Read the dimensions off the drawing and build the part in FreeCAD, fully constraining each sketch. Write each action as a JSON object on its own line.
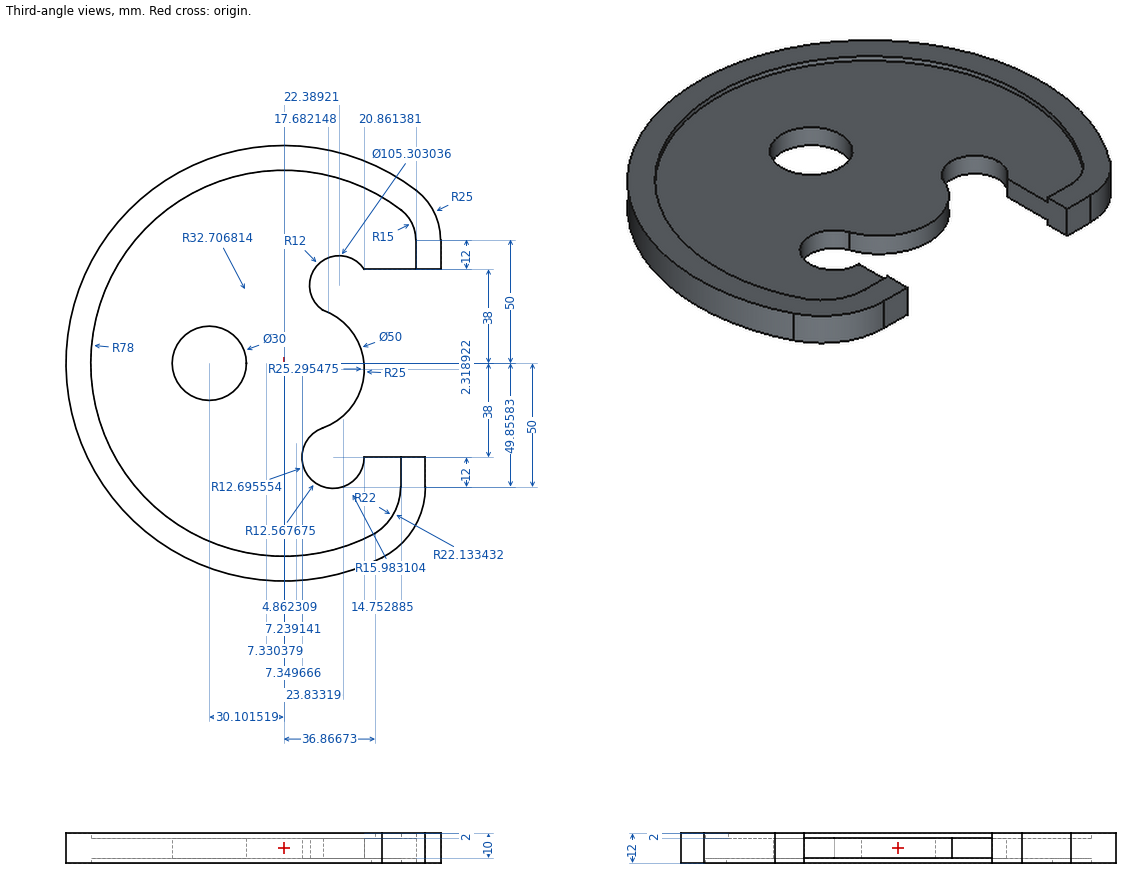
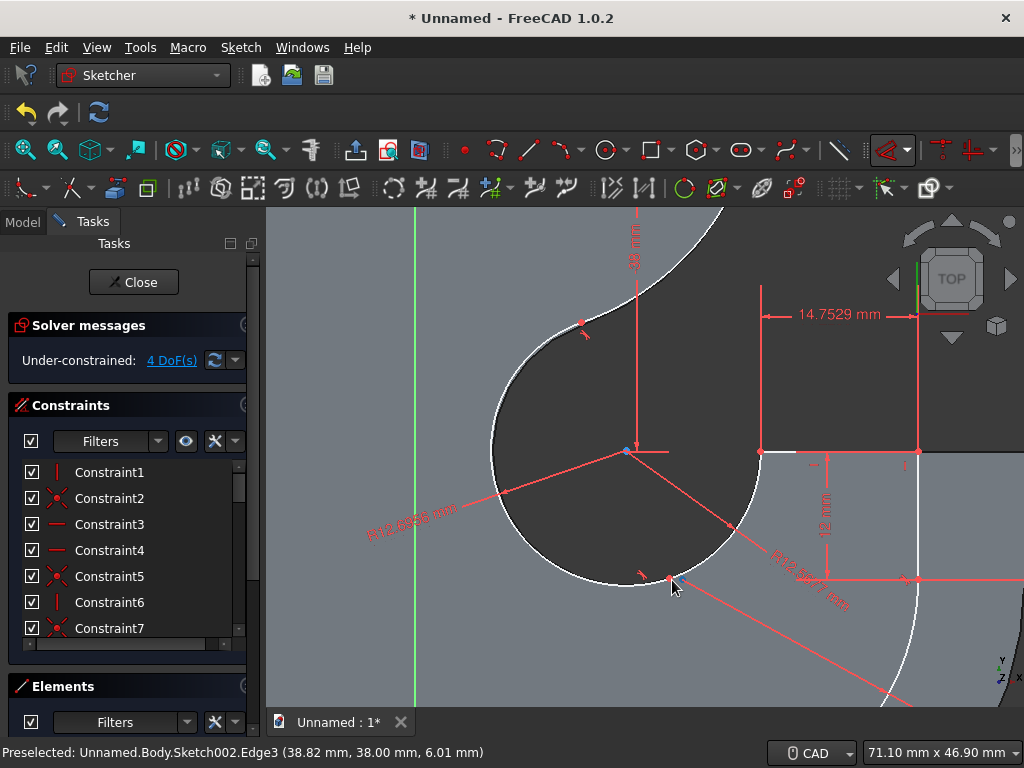
{"action": "left_click", "coordinate": [670, 579]}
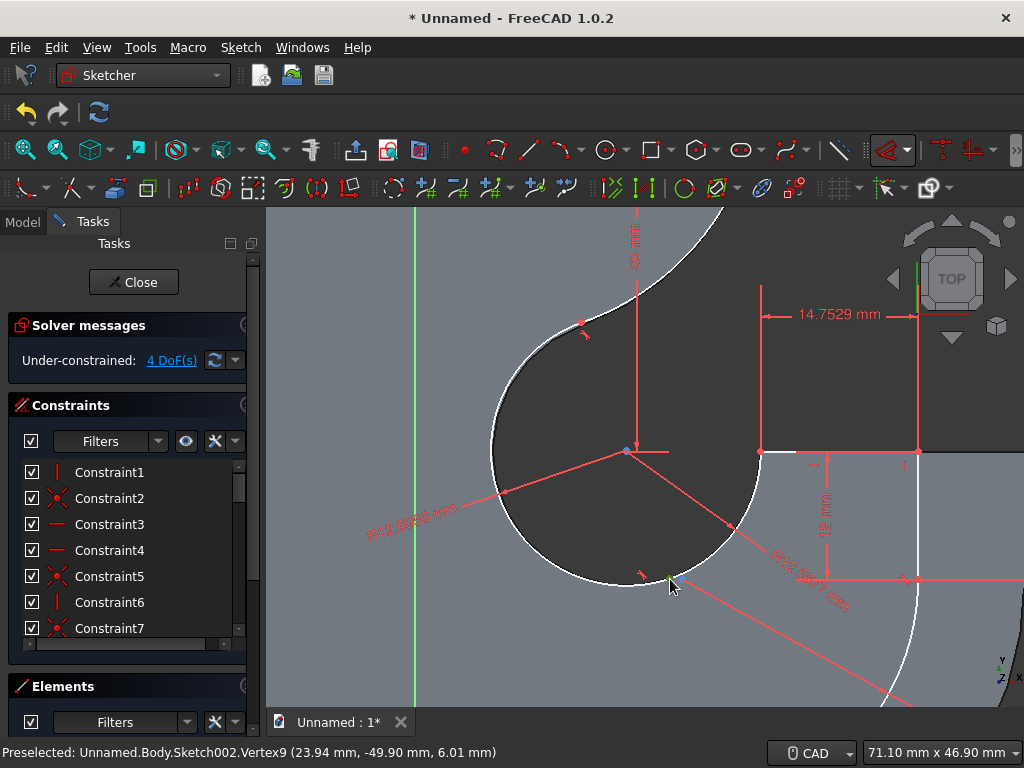
{"action": "key", "text": "i"}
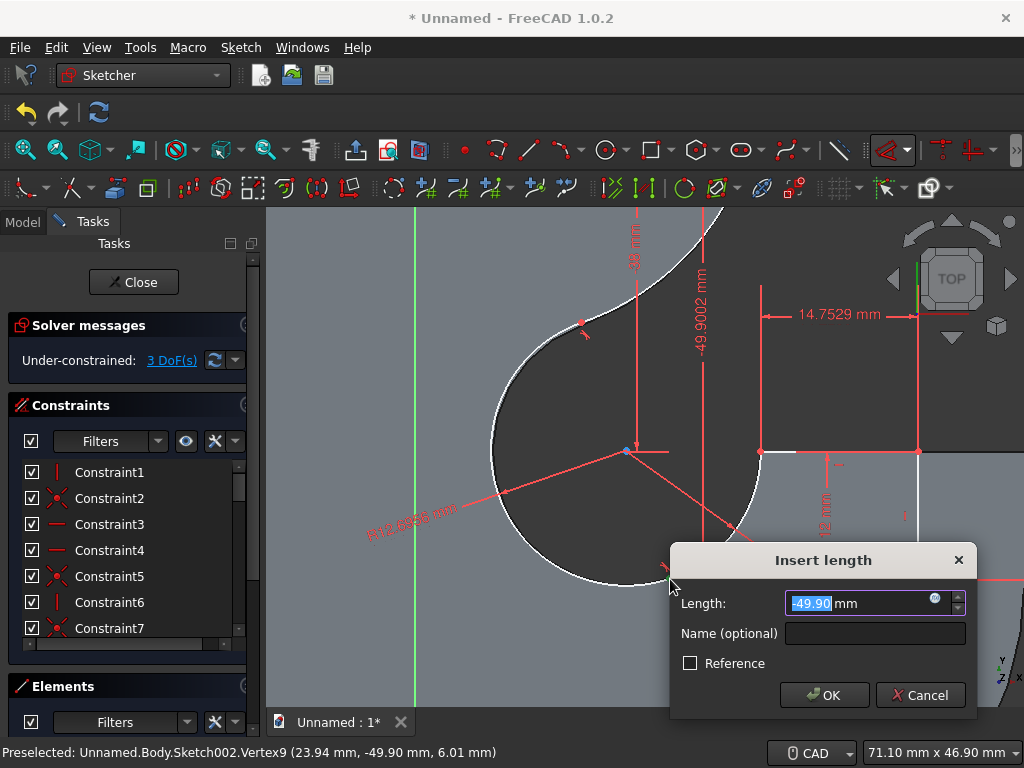
{"action": "type", "text": "-49.85583"}
{"action": "key", "text": "Return"}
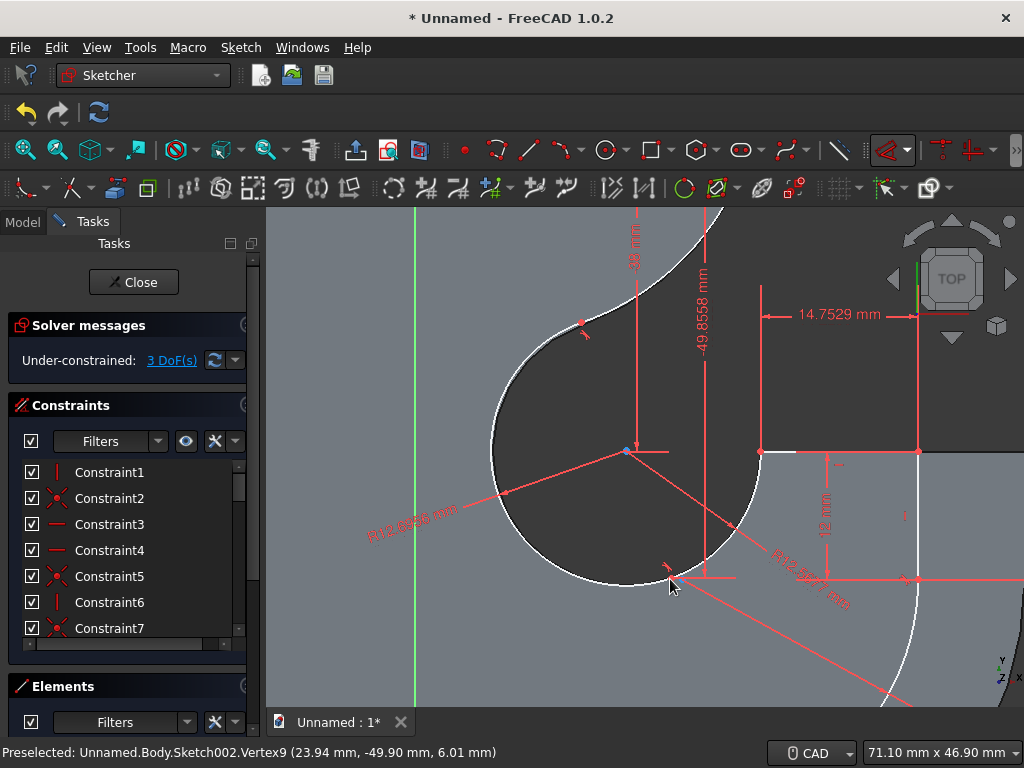
{"action": "scroll", "coordinate": [672, 579], "scroll_direction": "down", "scroll_amount": 7}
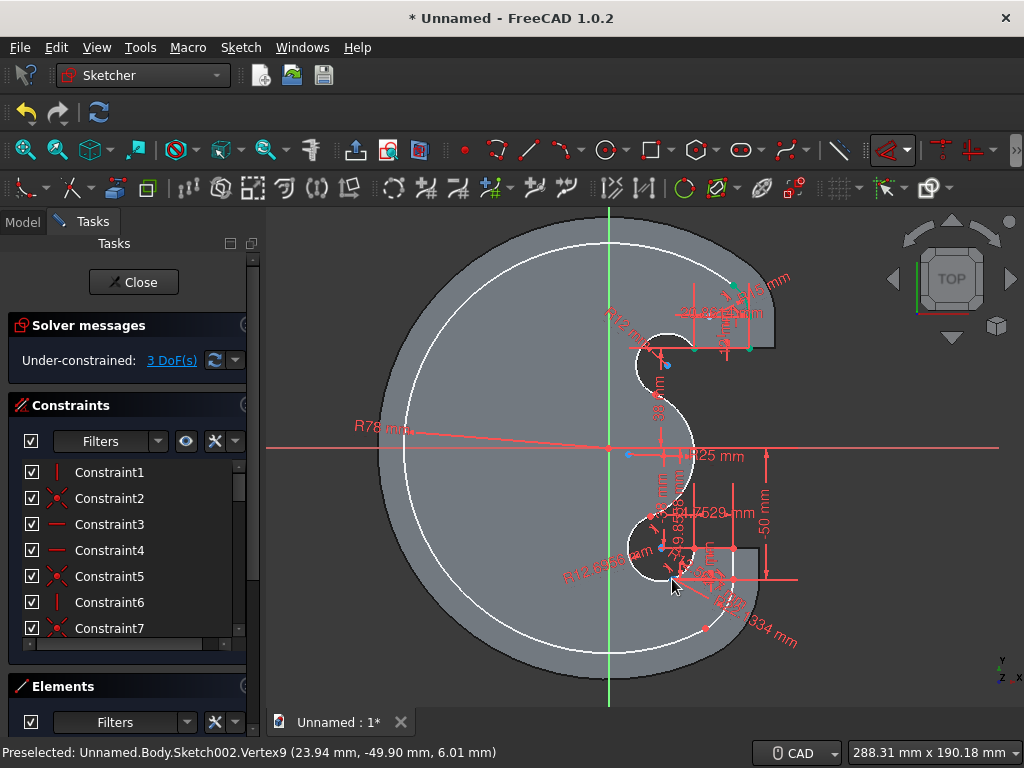
{"action": "left_click", "coordinate": [706, 629]}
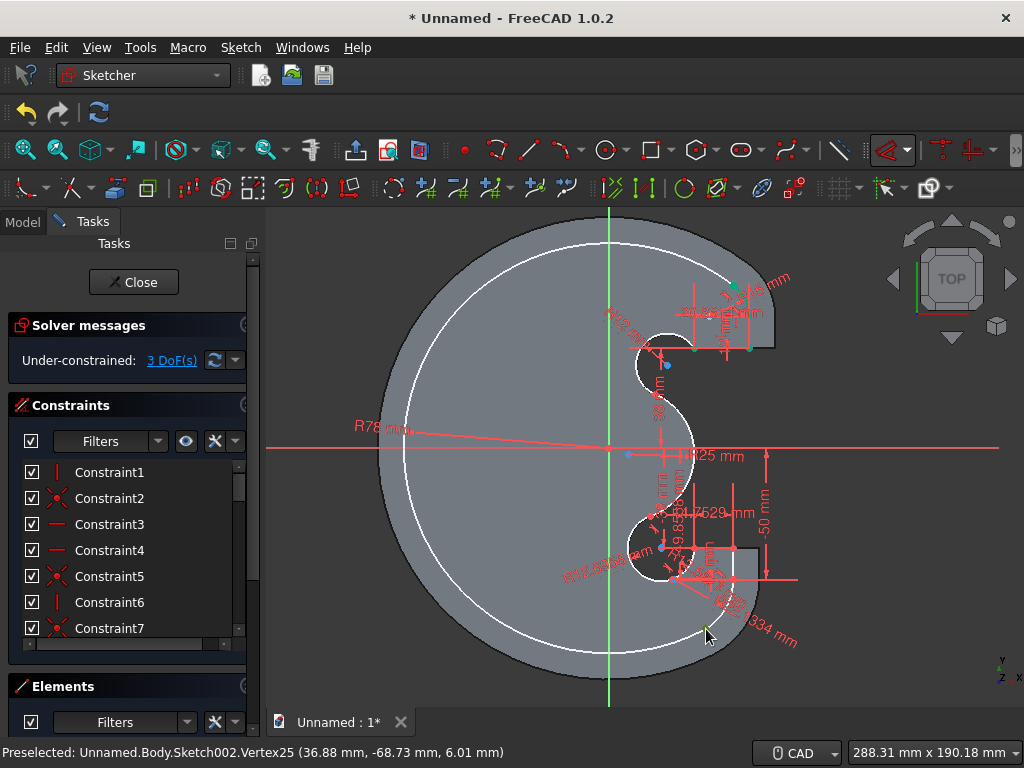
{"action": "key", "text": "l"}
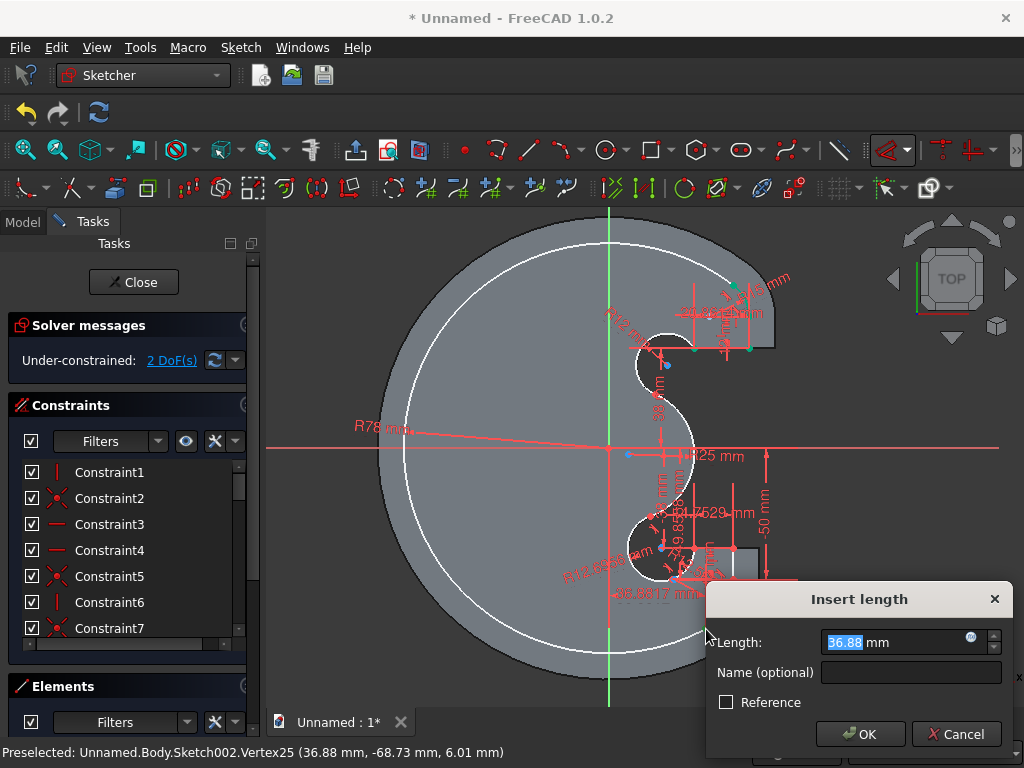
{"action": "type", "text": "36.86673"}
{"action": "key", "text": "Return"}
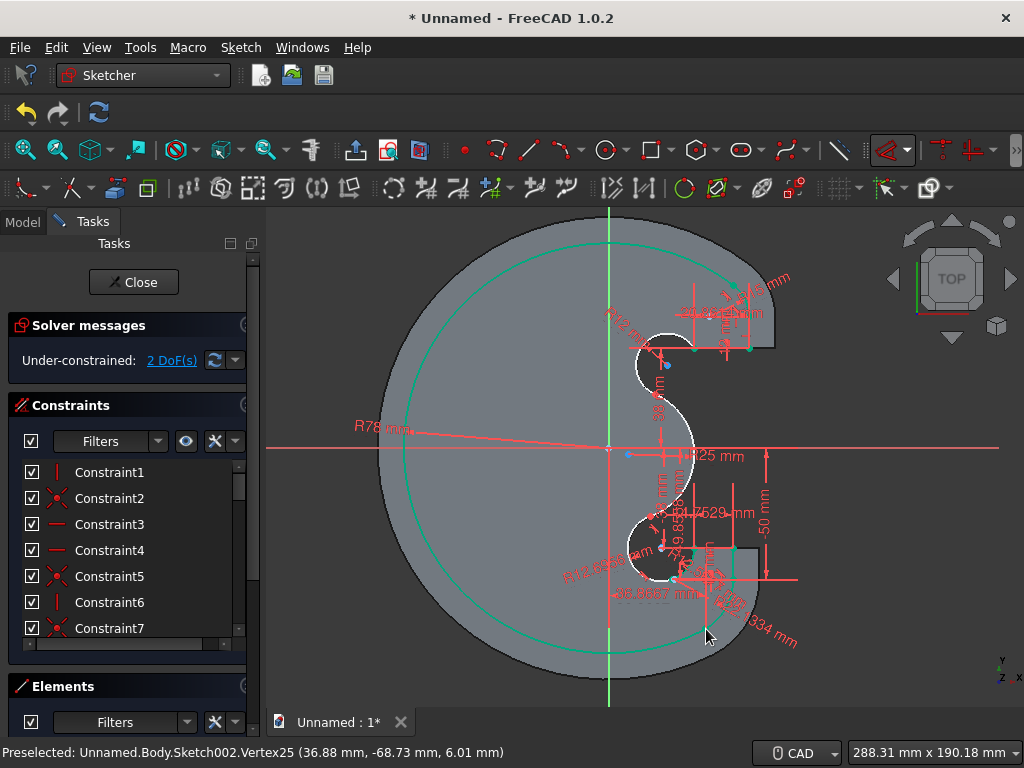
{"action": "scroll", "coordinate": [629, 454], "scroll_direction": "up", "scroll_amount": 4}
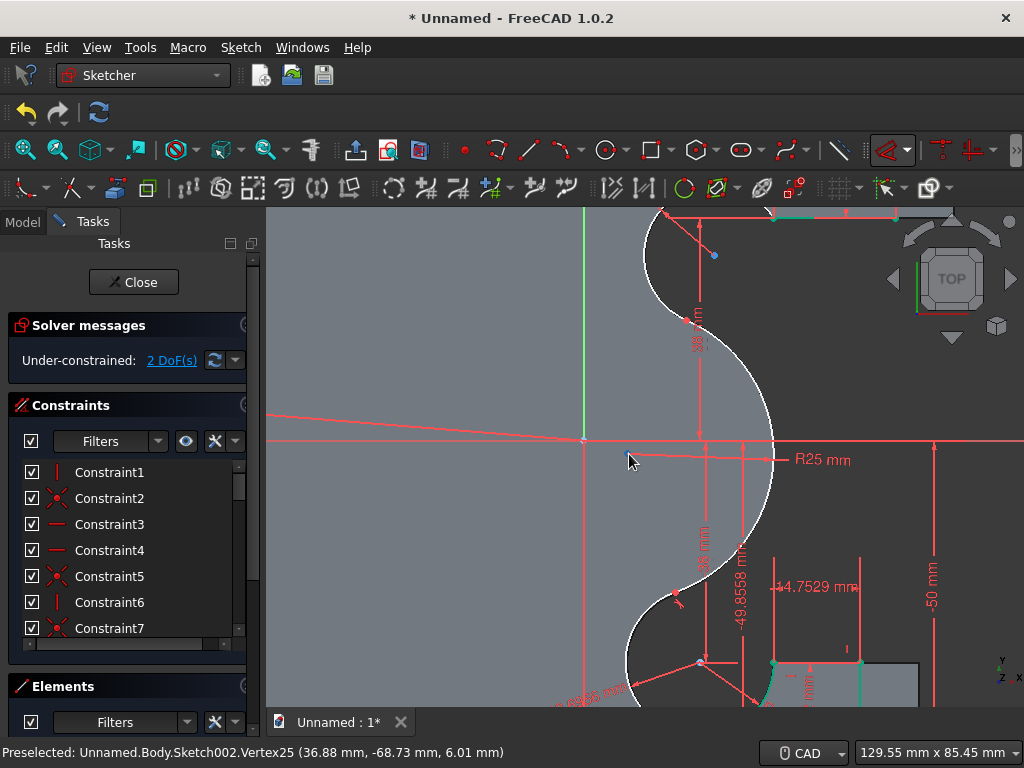
{"action": "left_click", "coordinate": [627, 454]}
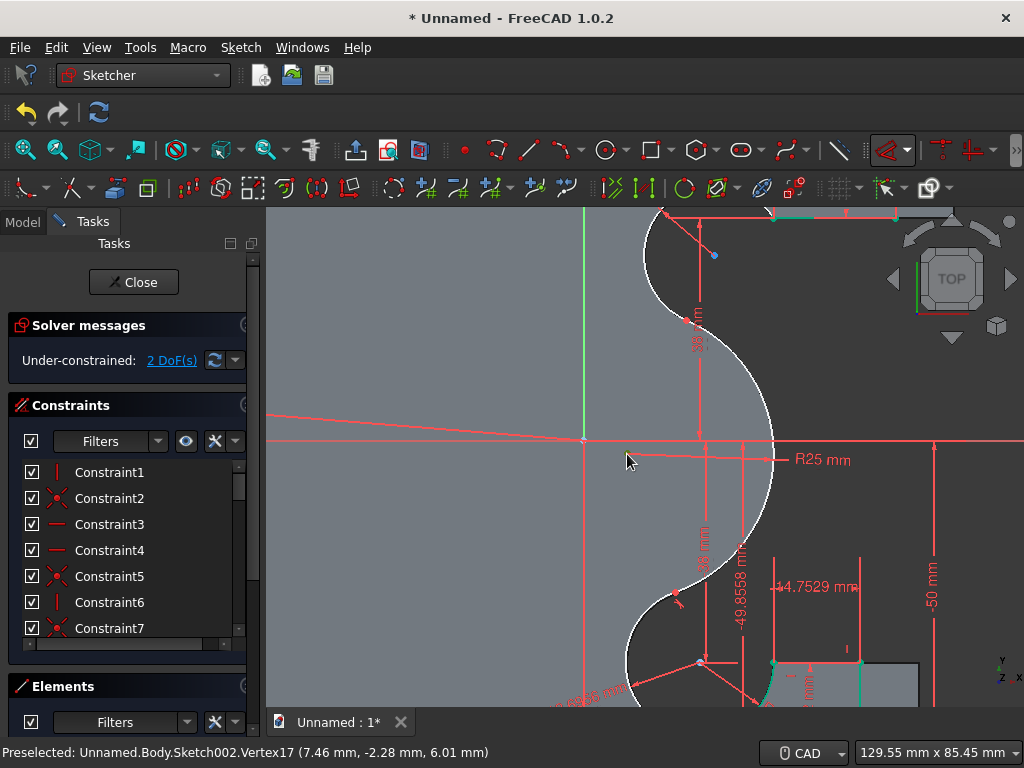
{"action": "left_click", "coordinate": [910, 150]}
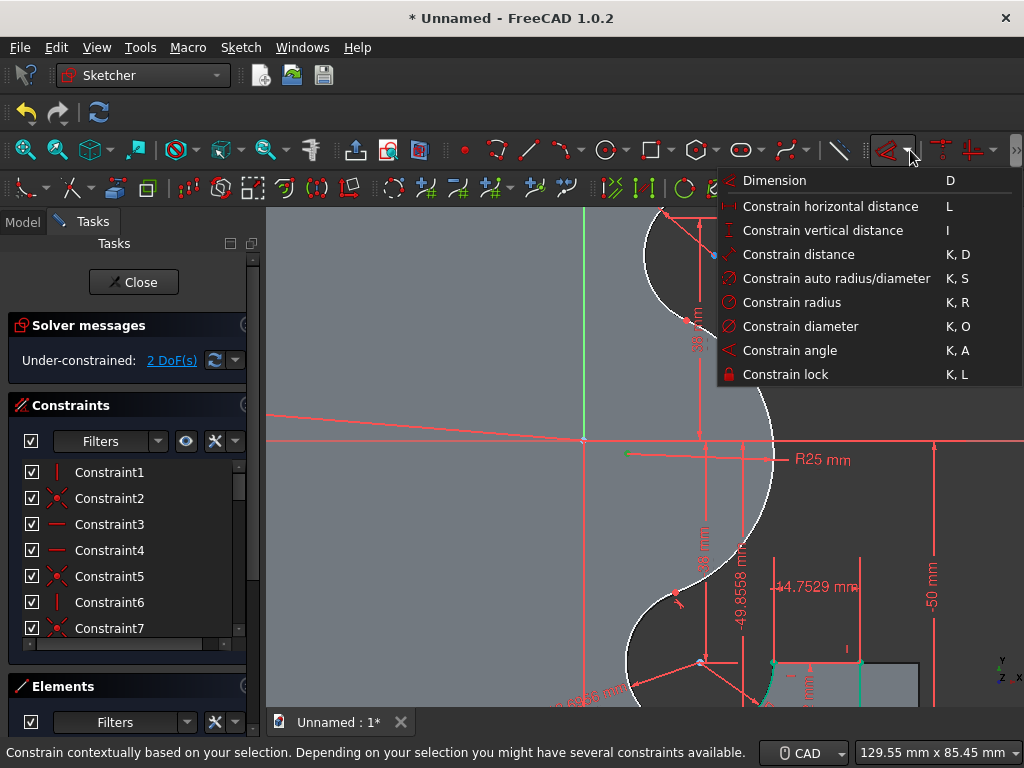
{"action": "left_click", "coordinate": [870, 206]}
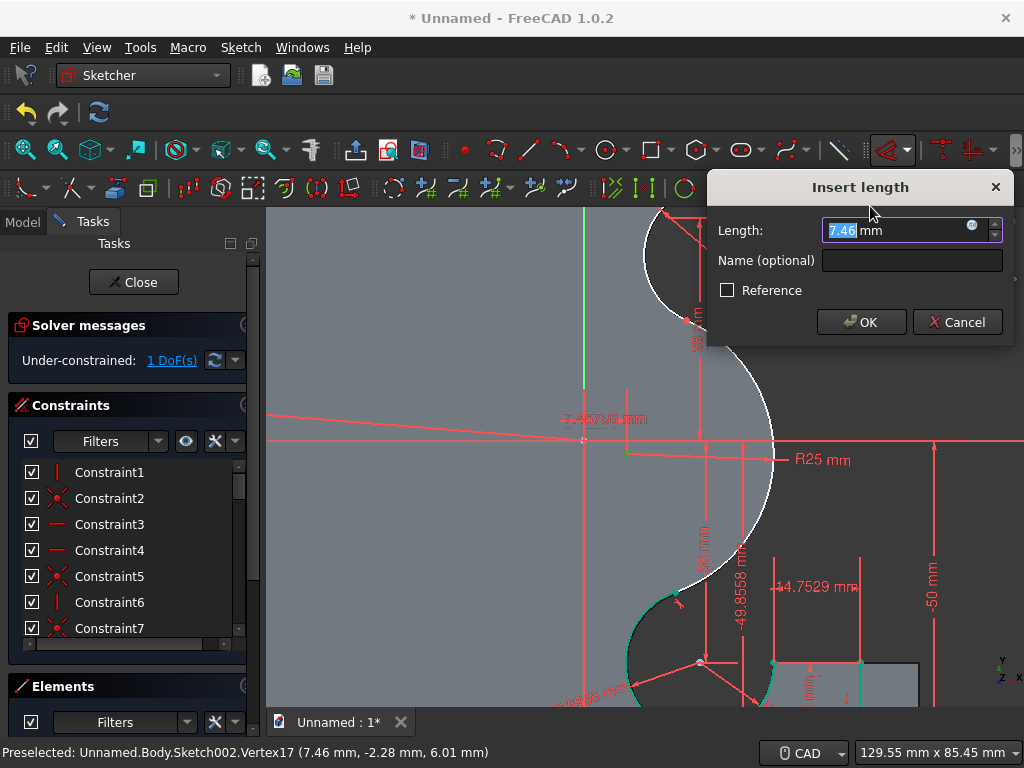
{"action": "type", "text": "7.349666"}
{"action": "key", "text": "Return"}